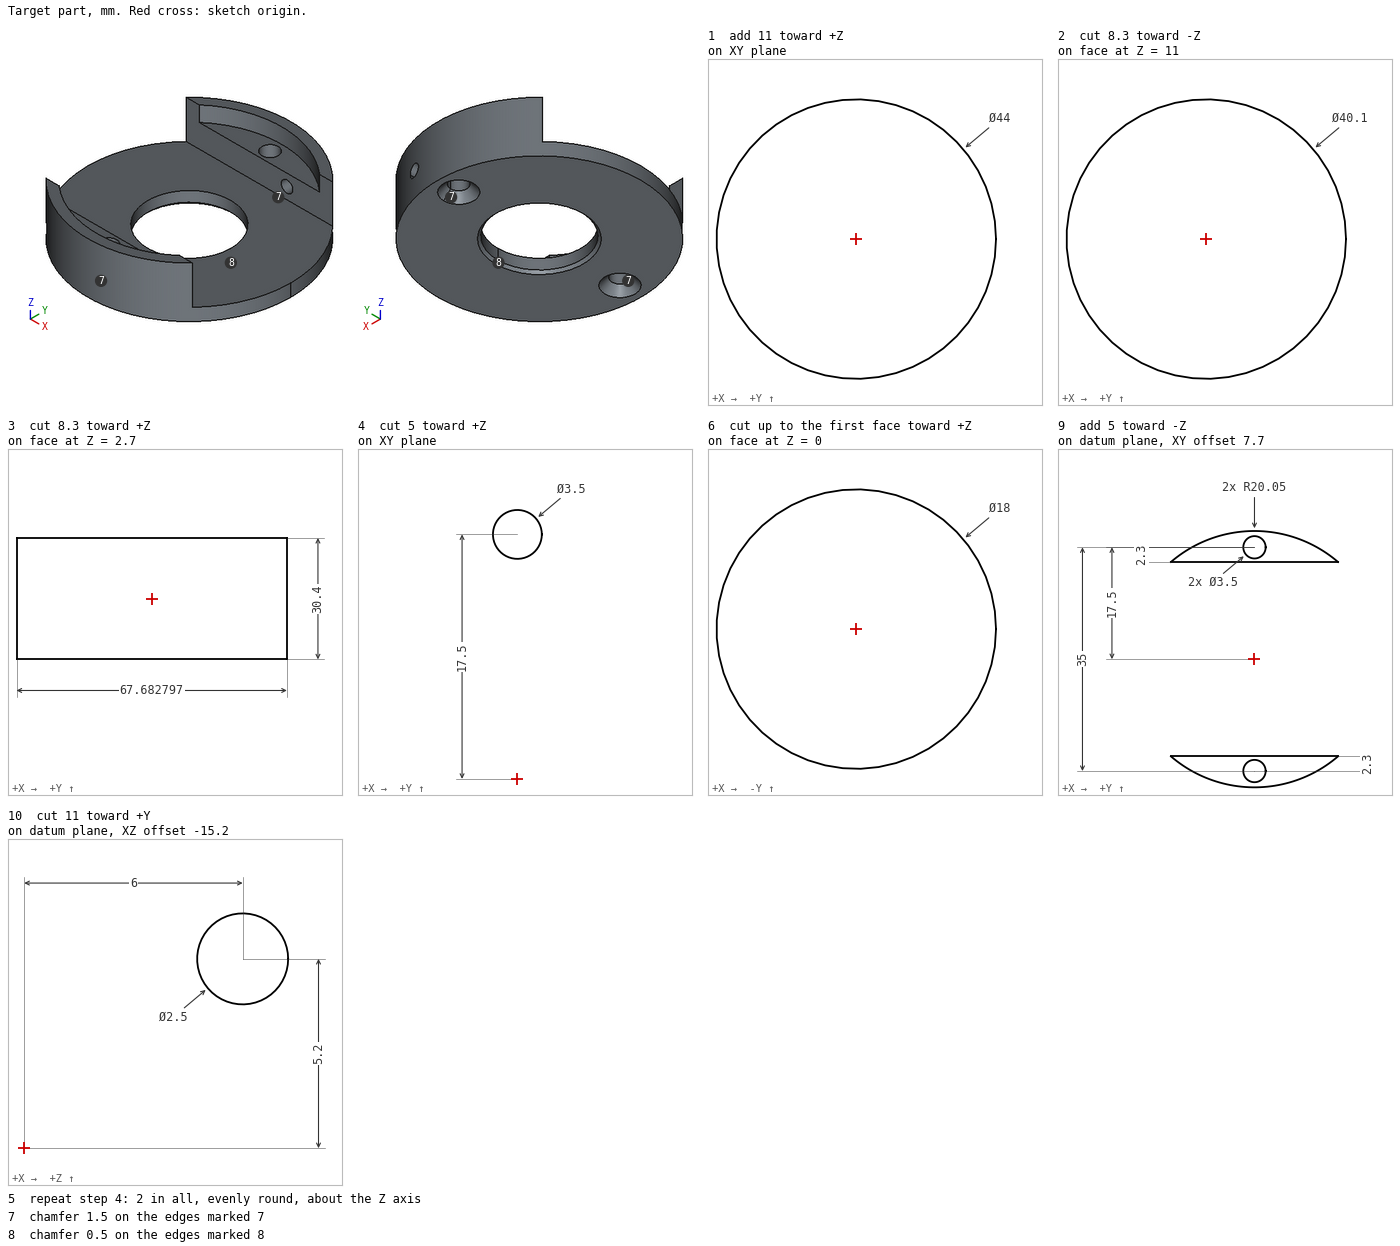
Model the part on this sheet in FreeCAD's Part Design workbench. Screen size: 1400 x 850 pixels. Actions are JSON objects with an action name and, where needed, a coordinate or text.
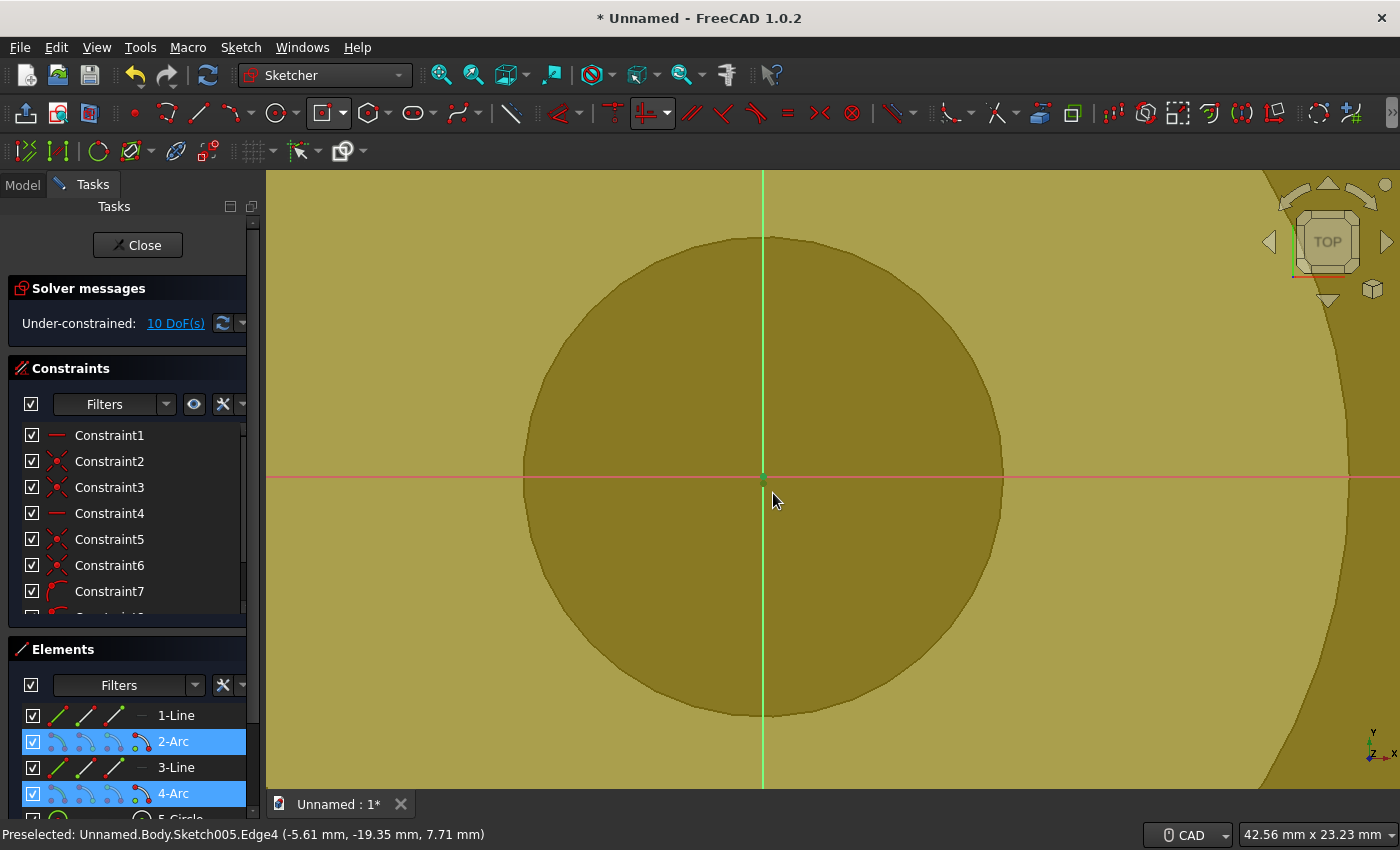
{"action": "left_click", "coordinate": [614, 114]}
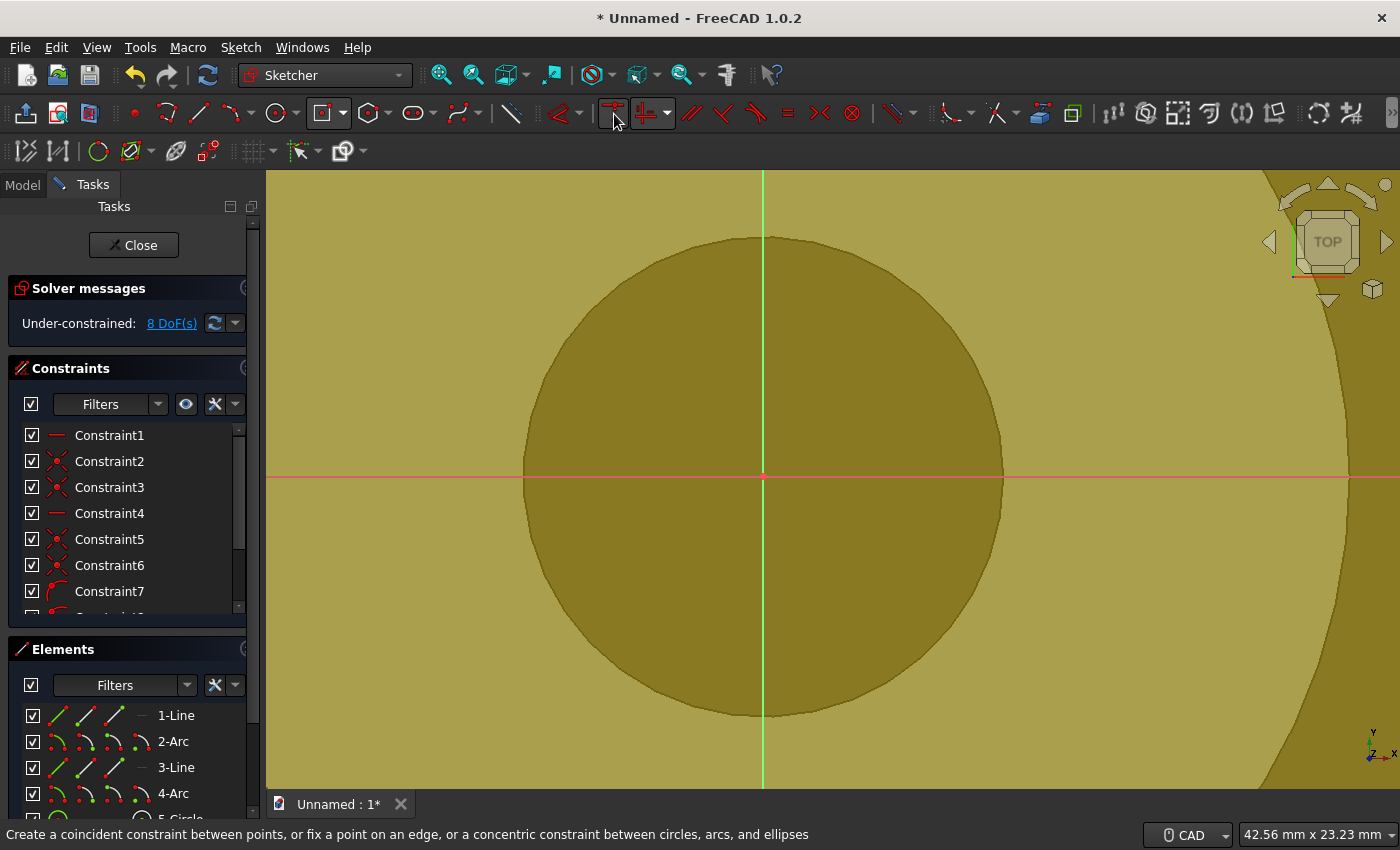
{"action": "scroll", "coordinate": [765, 481], "scroll_direction": "down", "scroll_amount": 5}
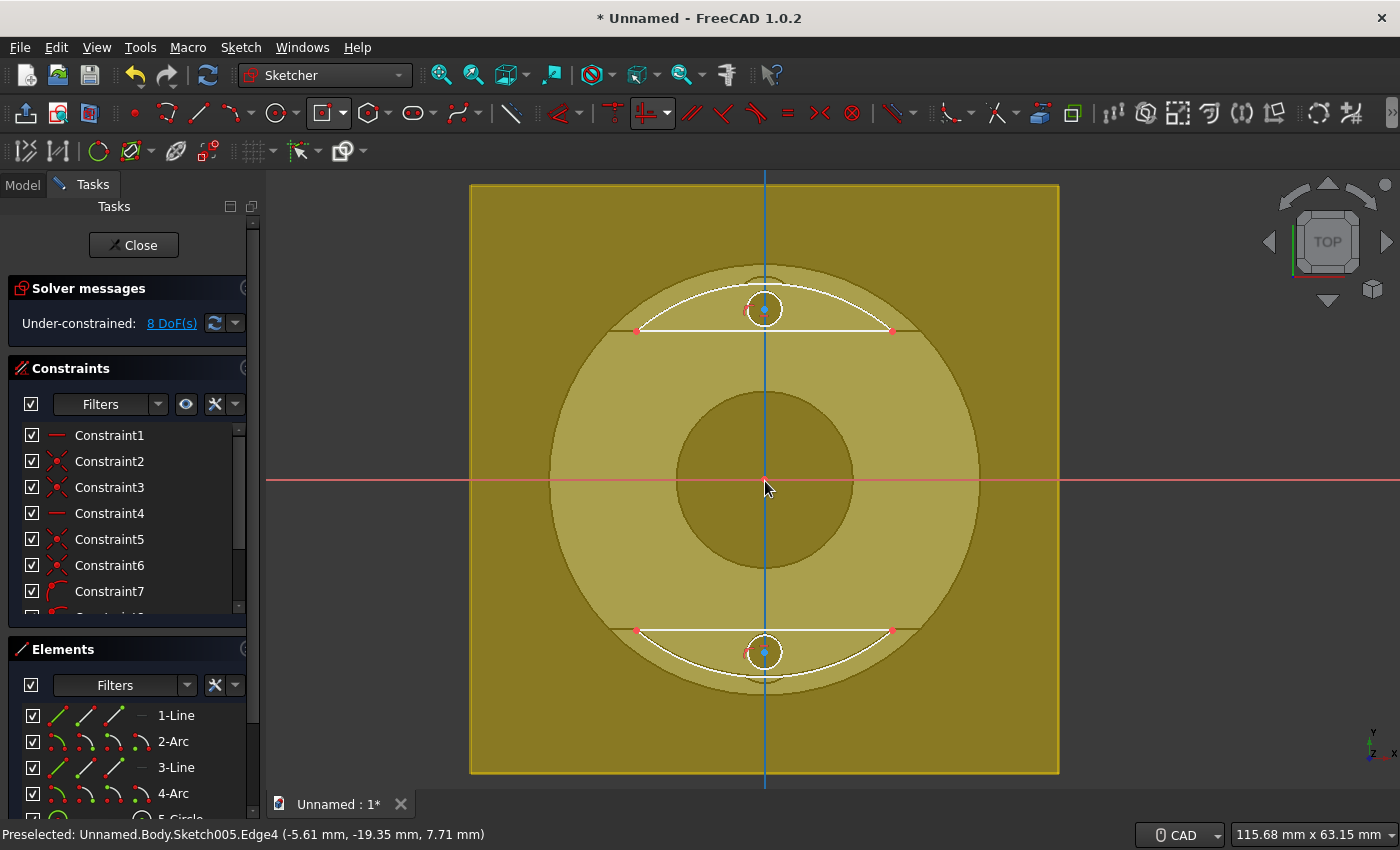
{"action": "left_click", "coordinate": [820, 292]}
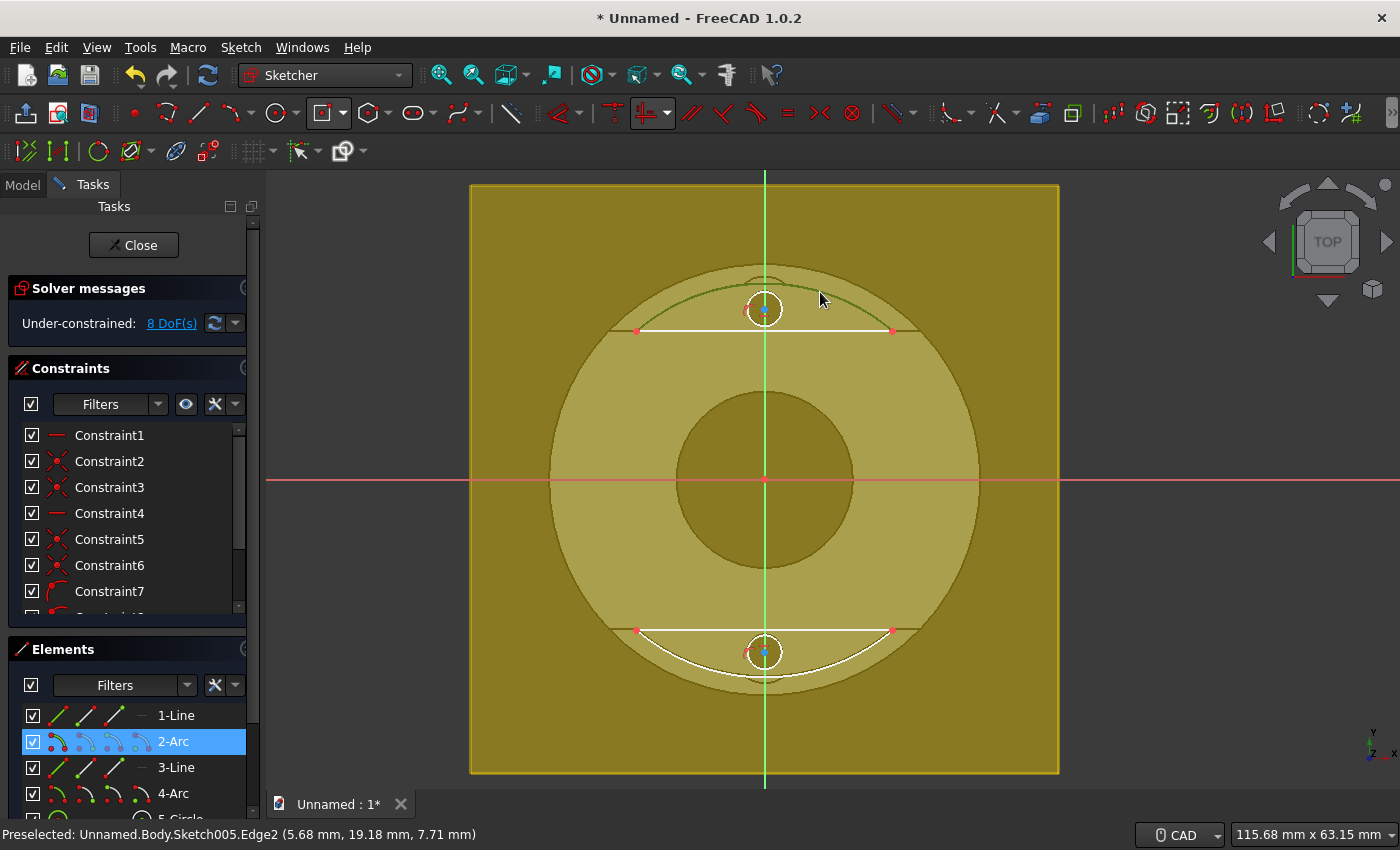
{"action": "left_click", "coordinate": [710, 670]}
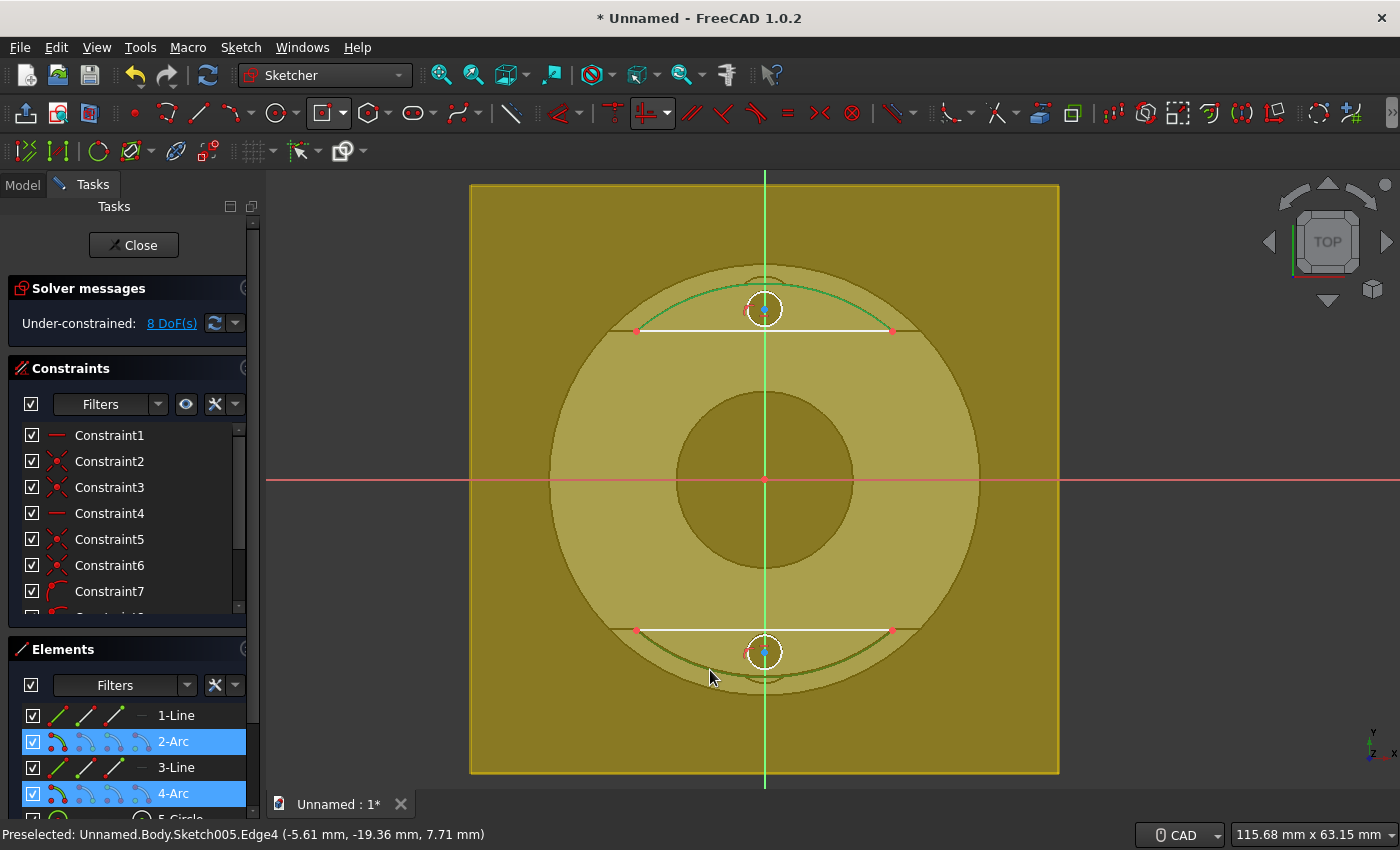
{"action": "key", "text": "e"}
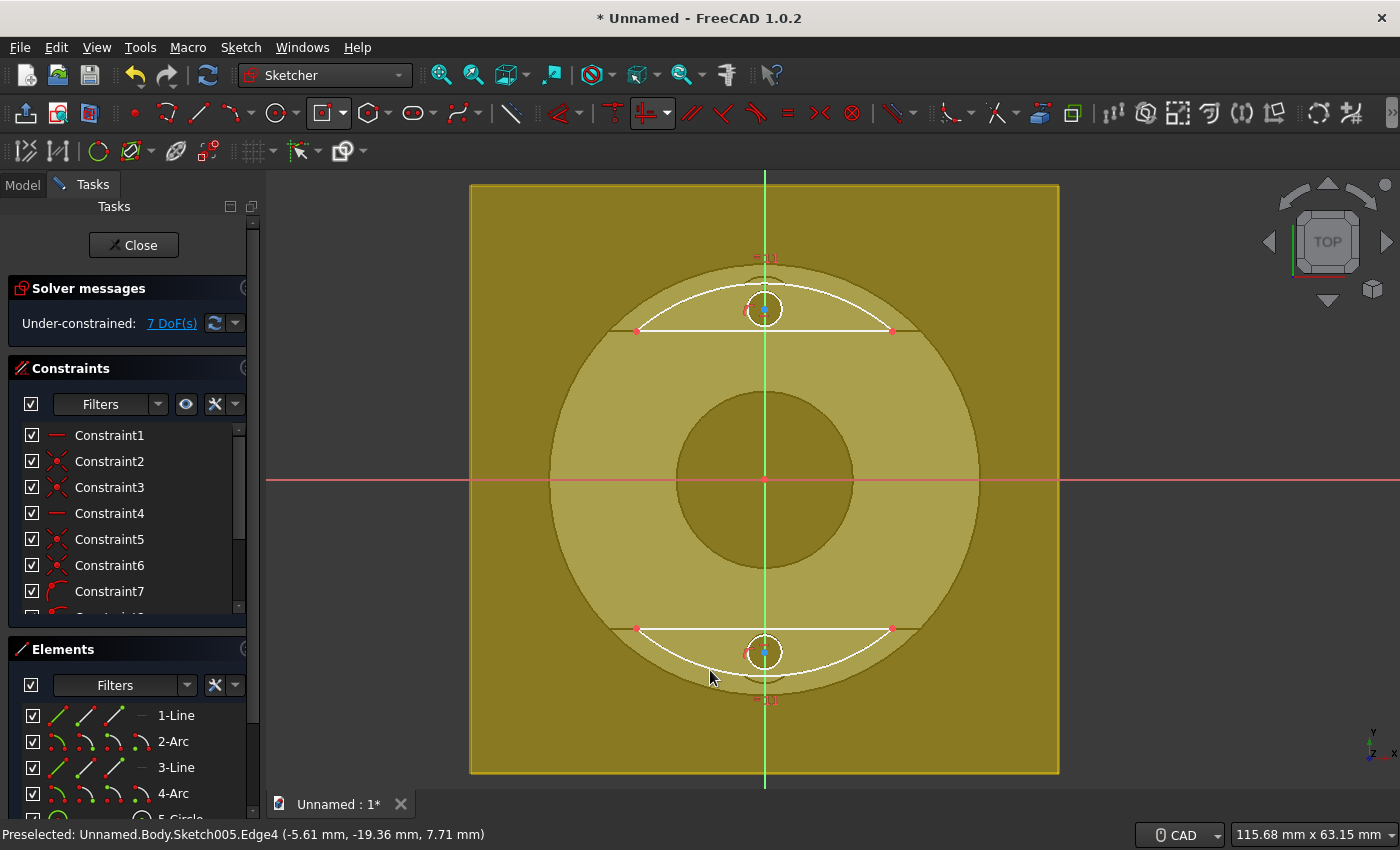
{"action": "left_click", "coordinate": [777, 297]}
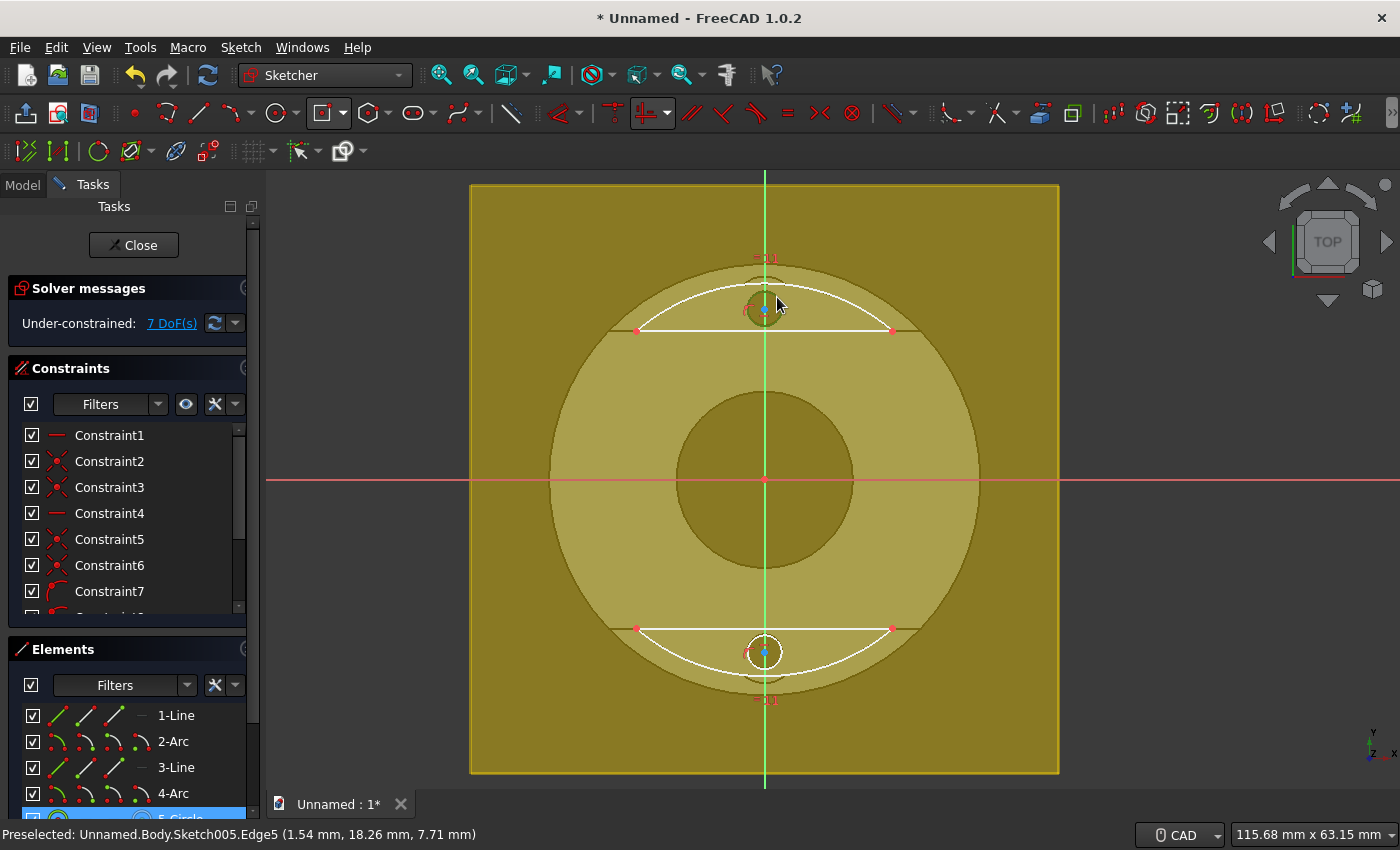
{"action": "left_click", "coordinate": [777, 640]}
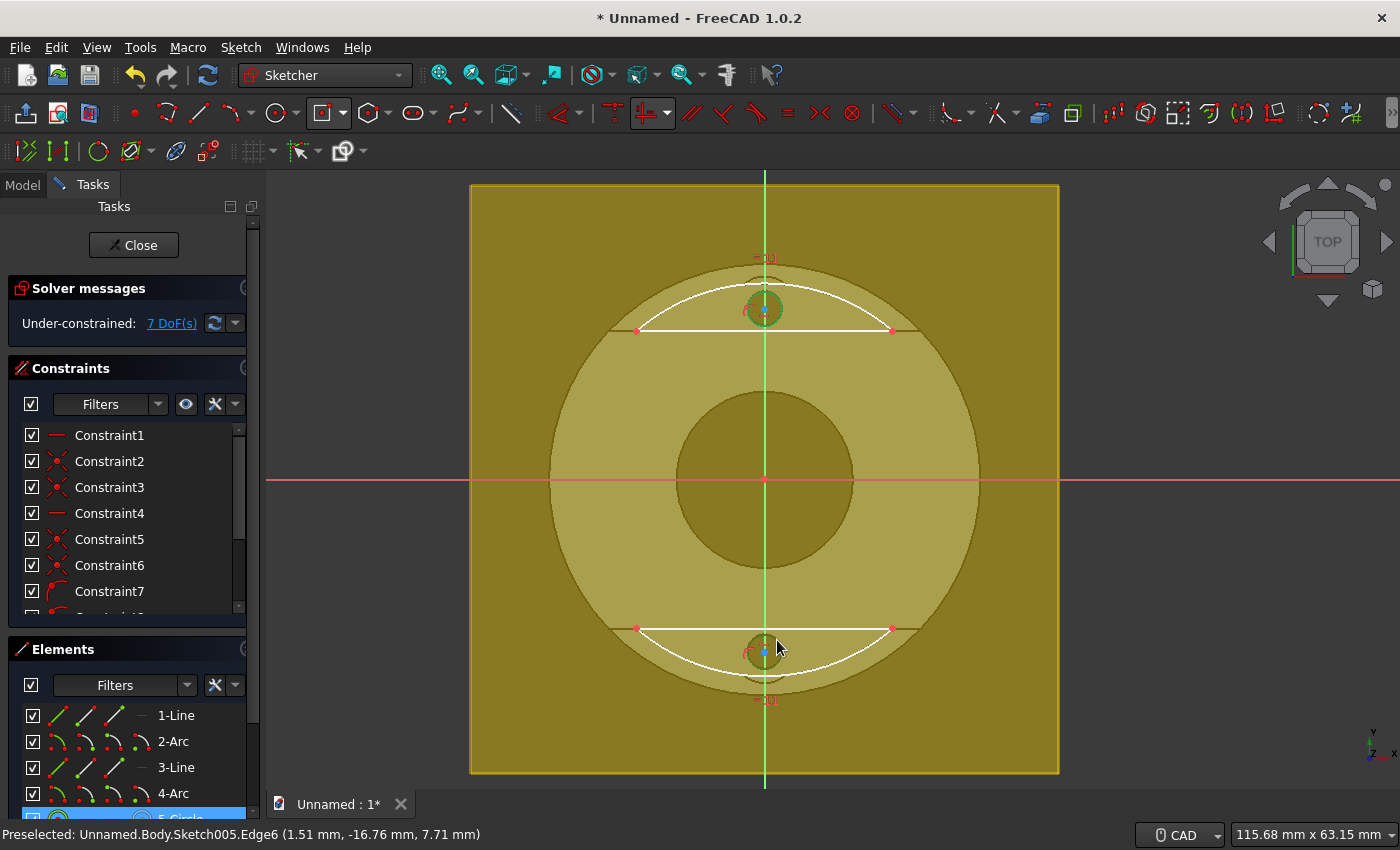
{"action": "key", "text": "e"}